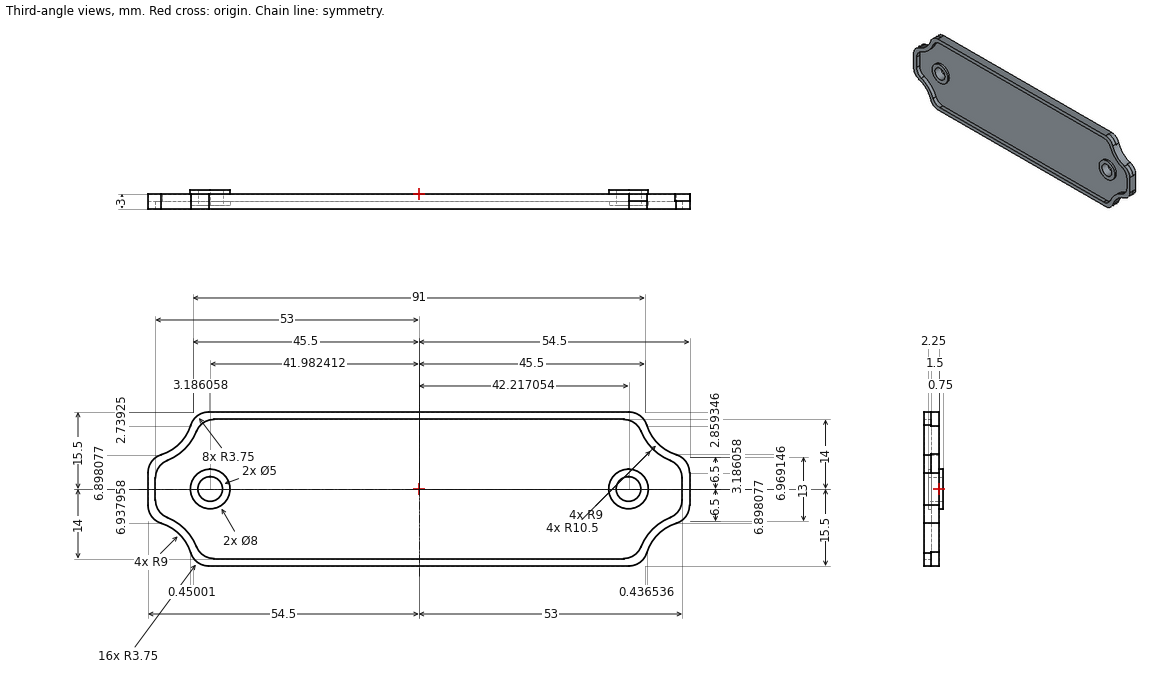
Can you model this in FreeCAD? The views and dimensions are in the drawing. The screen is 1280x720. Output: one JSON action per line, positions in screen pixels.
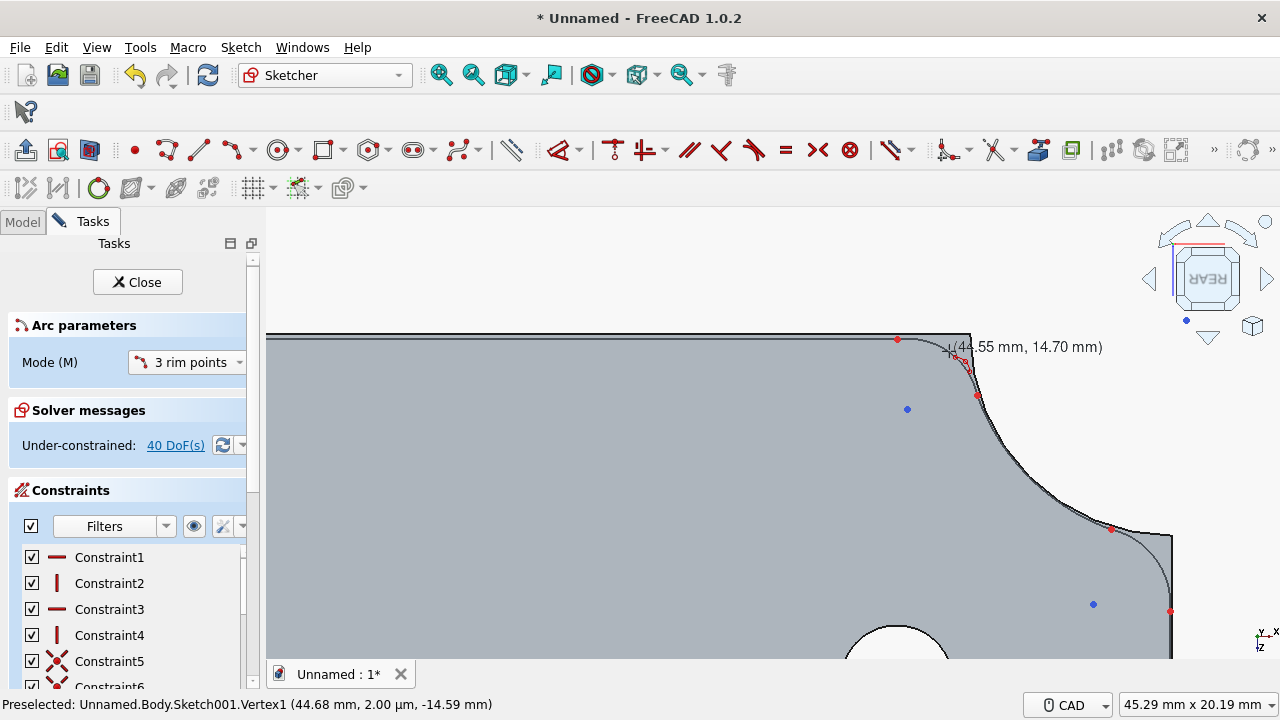
{"action": "left_click", "coordinate": [200, 150]}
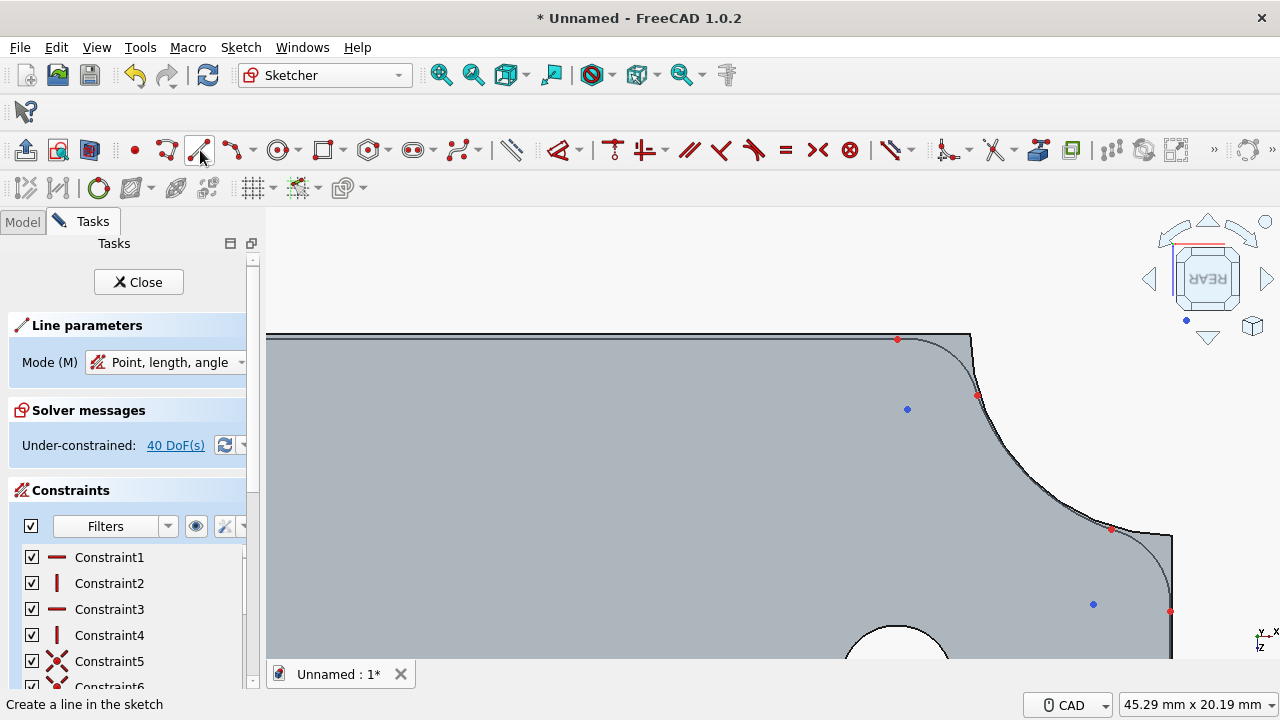
{"action": "scroll", "coordinate": [951, 352], "scroll_direction": "down", "scroll_amount": 7}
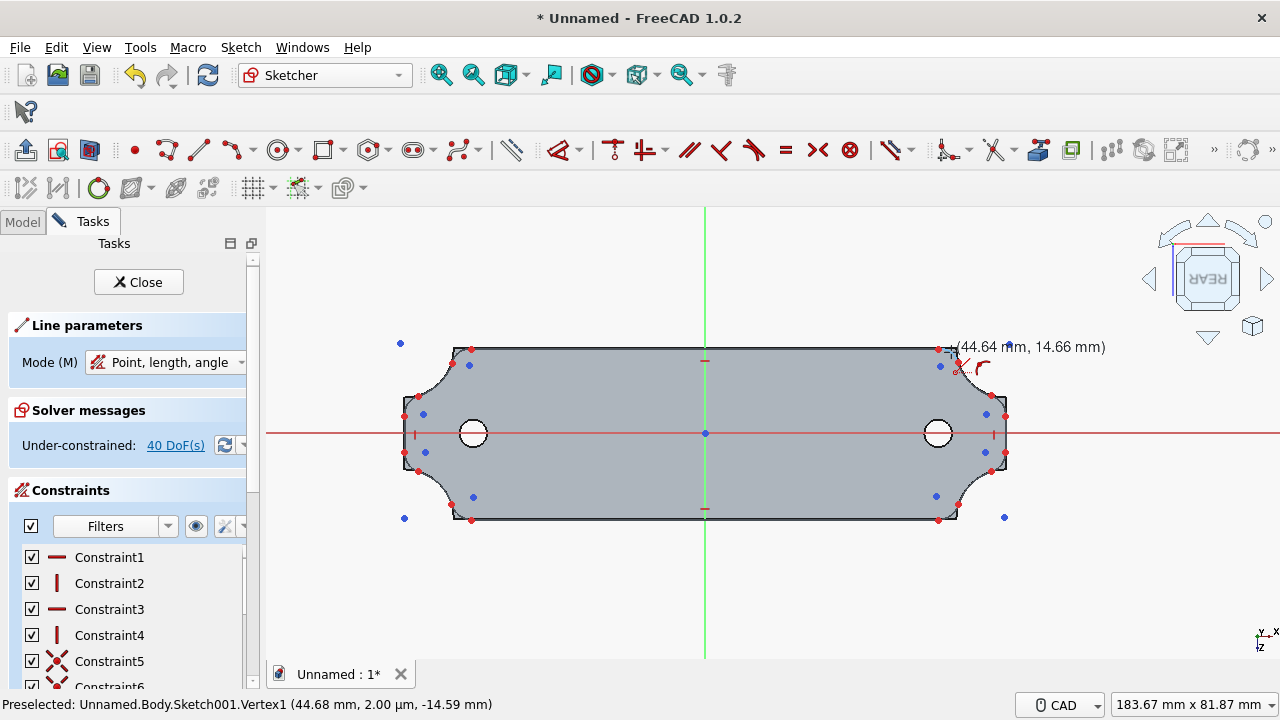
{"action": "scroll", "coordinate": [998, 421], "scroll_direction": "up", "scroll_amount": 4}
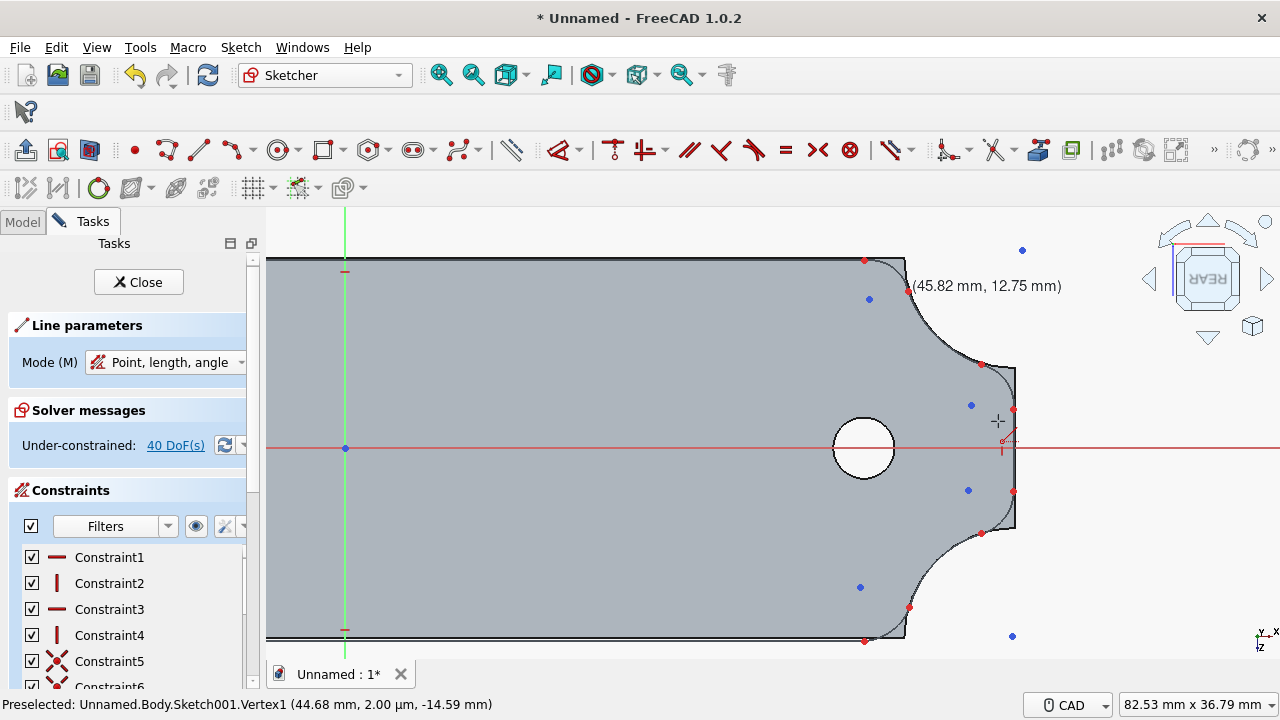
{"action": "left_click", "coordinate": [996, 420]}
{"action": "left_click", "coordinate": [996, 476]}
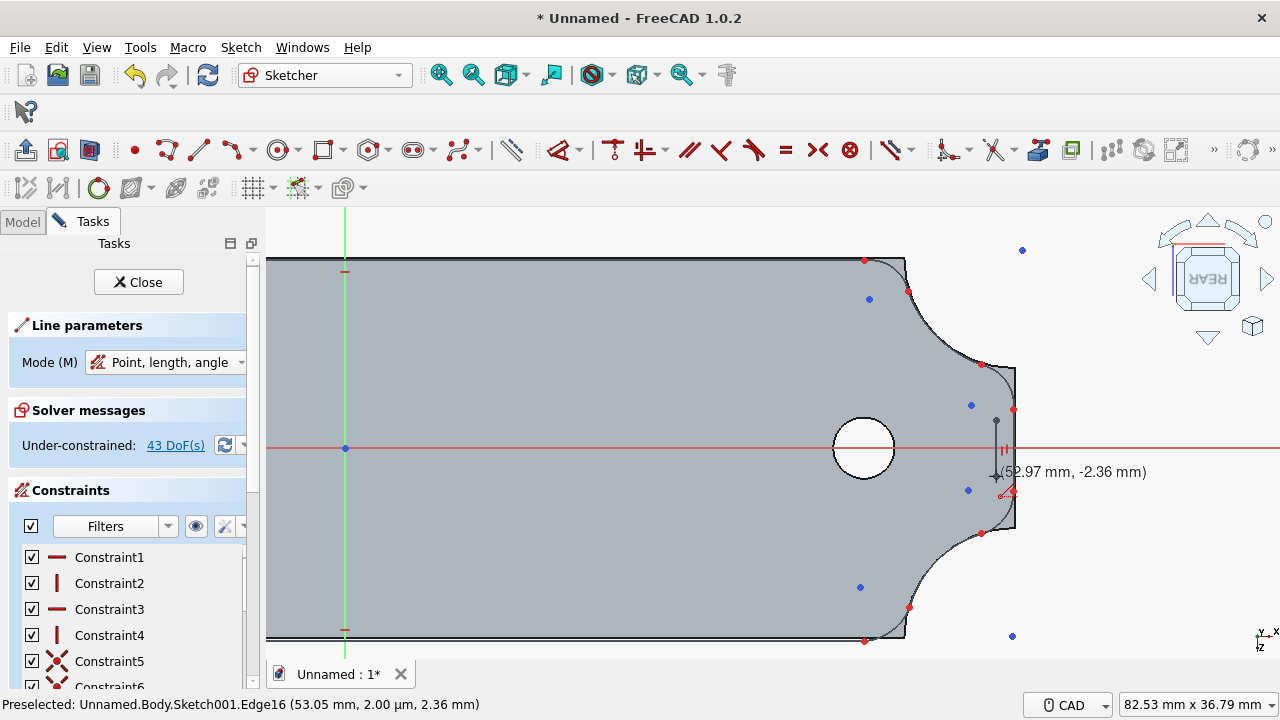
{"action": "left_click", "coordinate": [852, 620]}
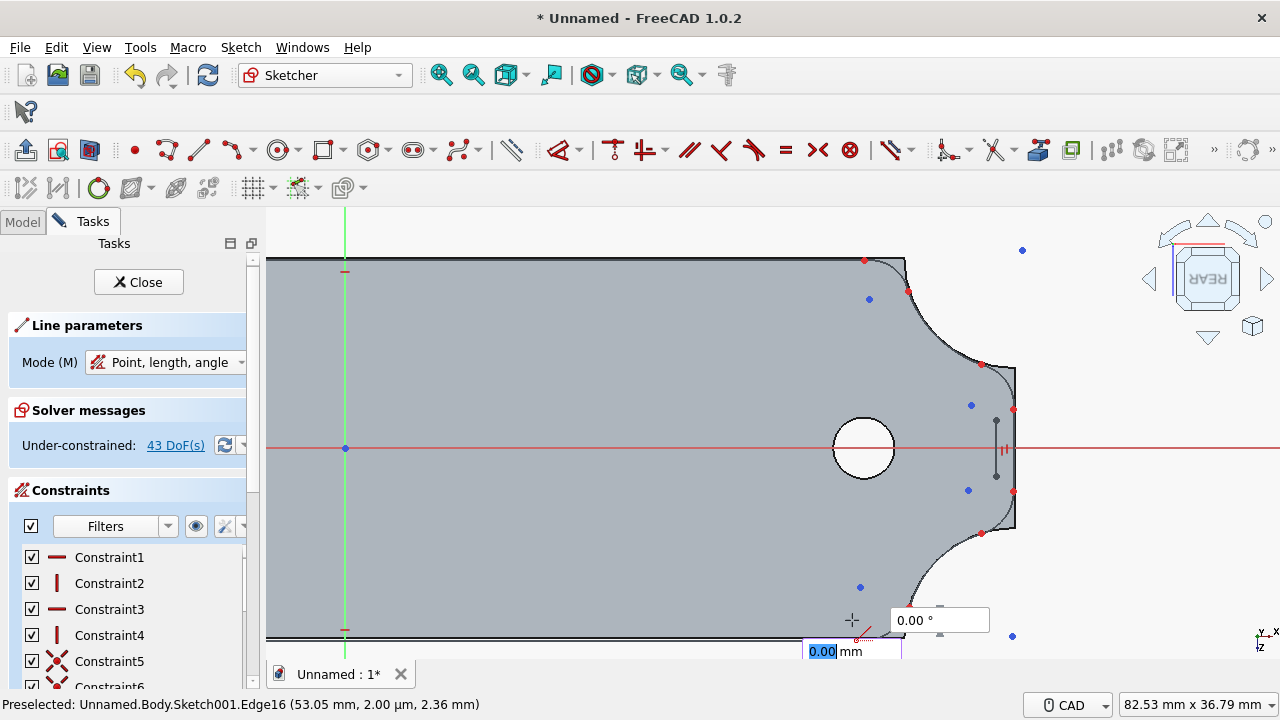
{"action": "scroll", "coordinate": [998, 421], "scroll_direction": "down", "scroll_amount": 4}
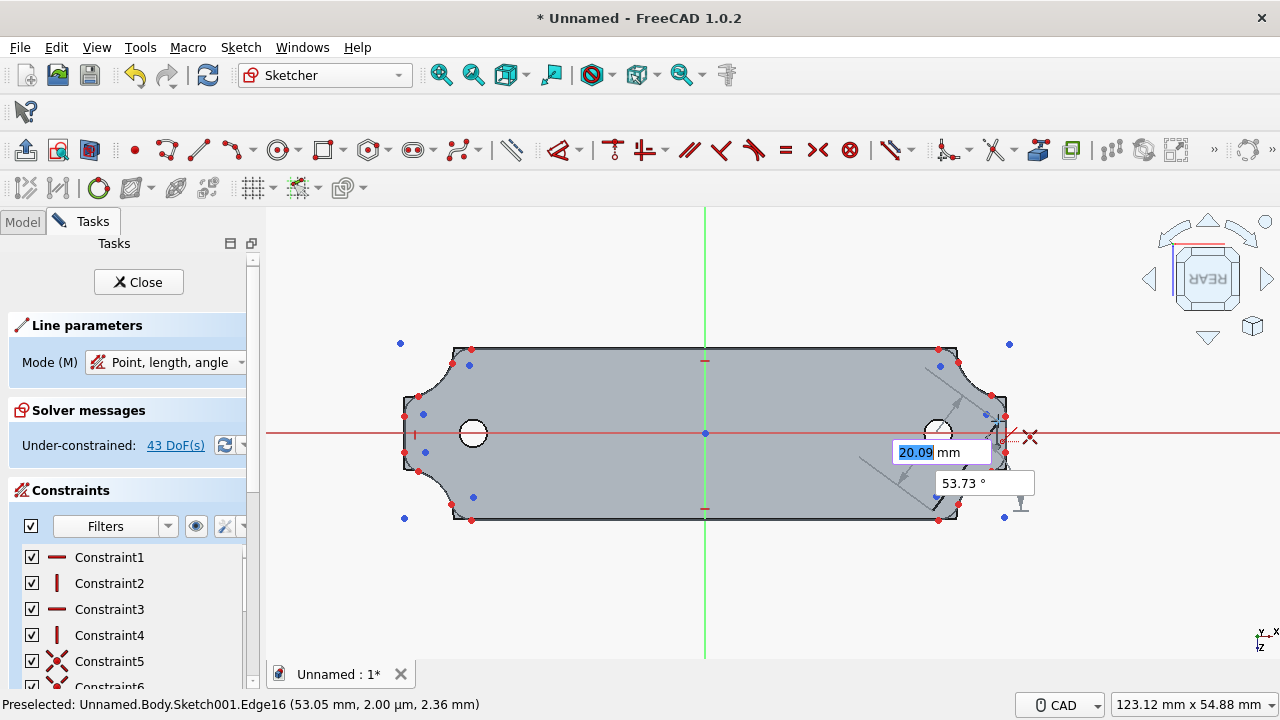
{"action": "scroll", "coordinate": [477, 511], "scroll_direction": "up", "scroll_amount": 4}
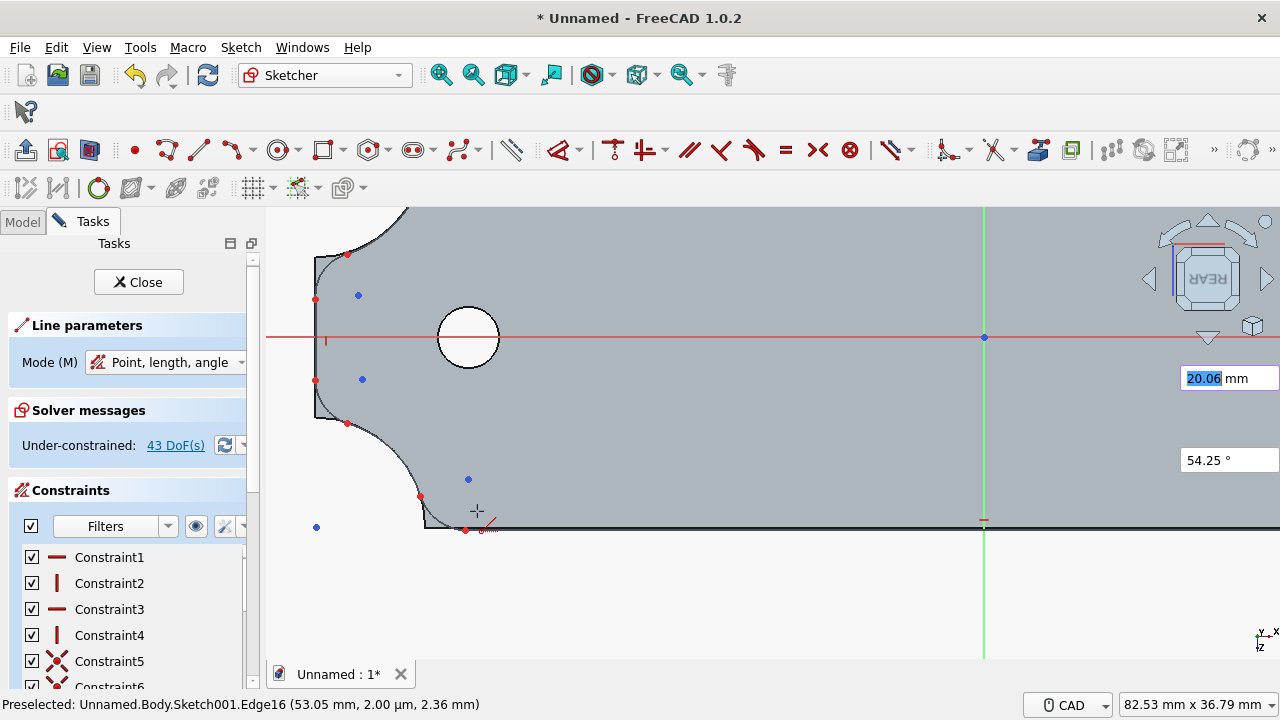
{"action": "left_click", "coordinate": [477, 509]}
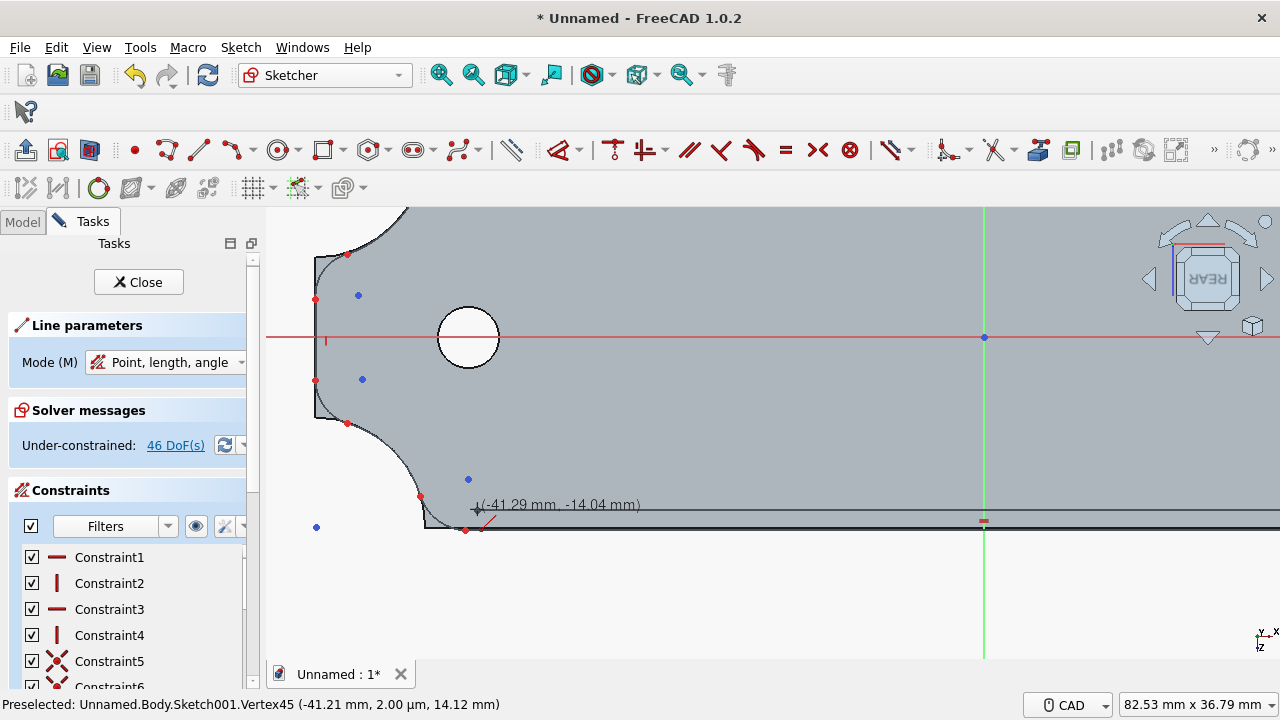
{"action": "left_click", "coordinate": [333, 365]}
{"action": "left_click", "coordinate": [333, 310]}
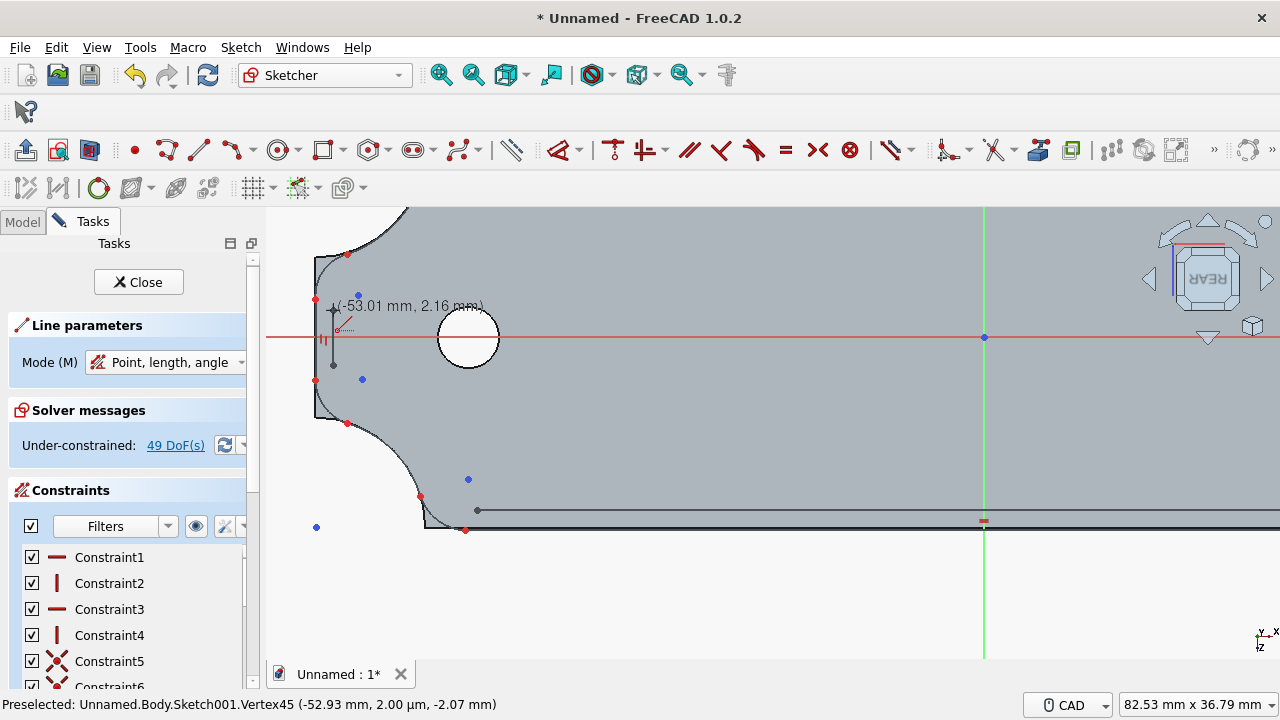
{"action": "scroll", "coordinate": [476, 511], "scroll_direction": "down", "scroll_amount": 4}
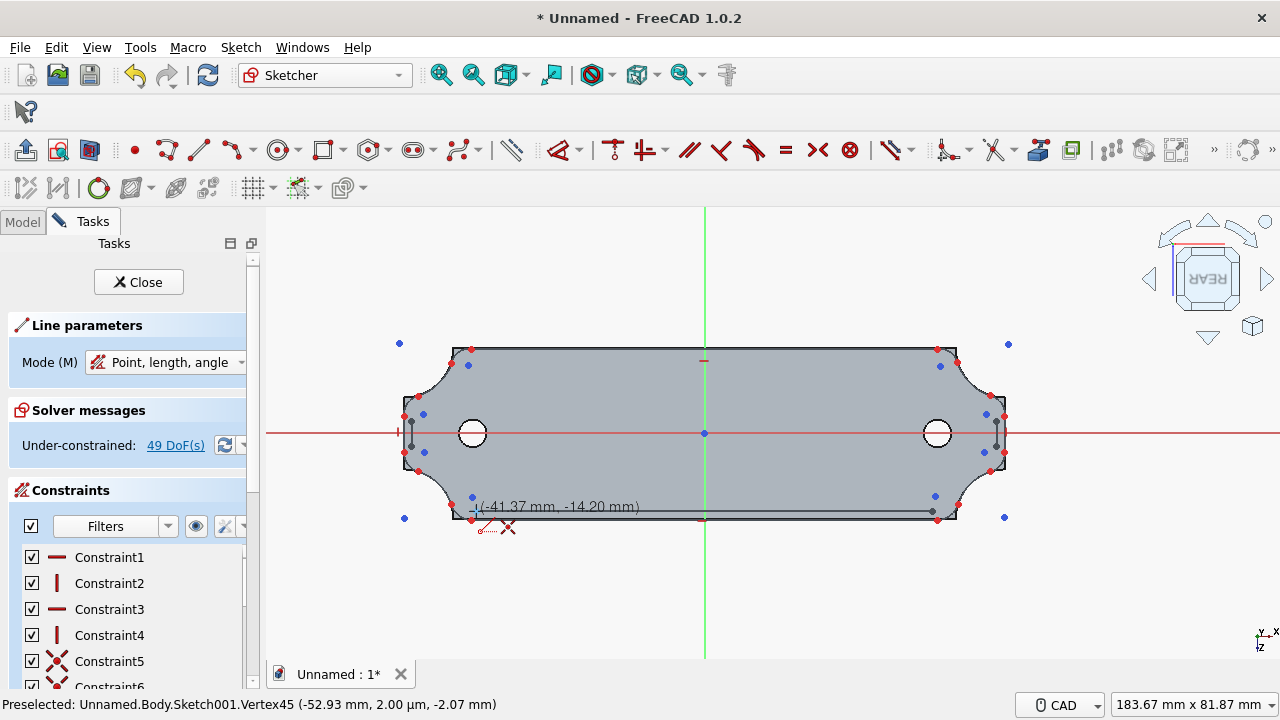
{"action": "scroll", "coordinate": [477, 356], "scroll_direction": "up", "scroll_amount": 4}